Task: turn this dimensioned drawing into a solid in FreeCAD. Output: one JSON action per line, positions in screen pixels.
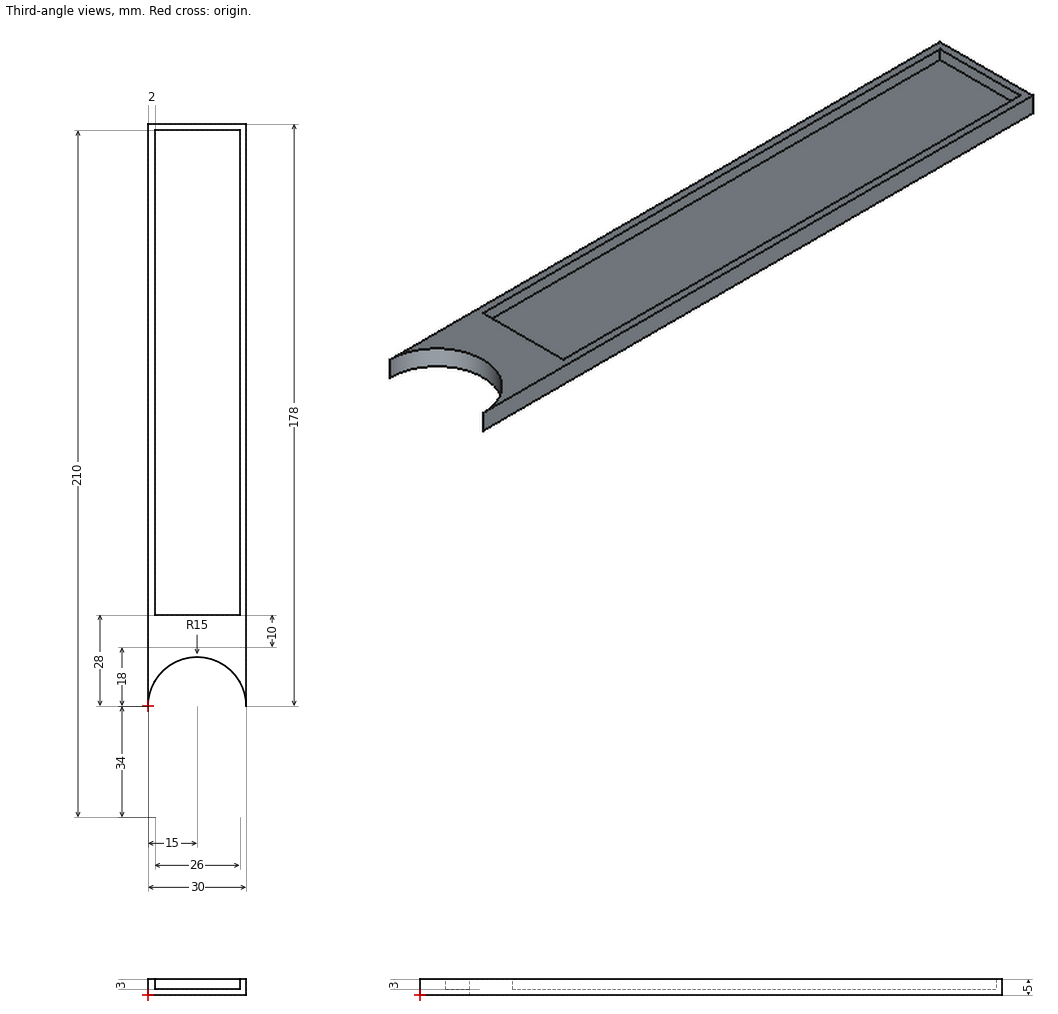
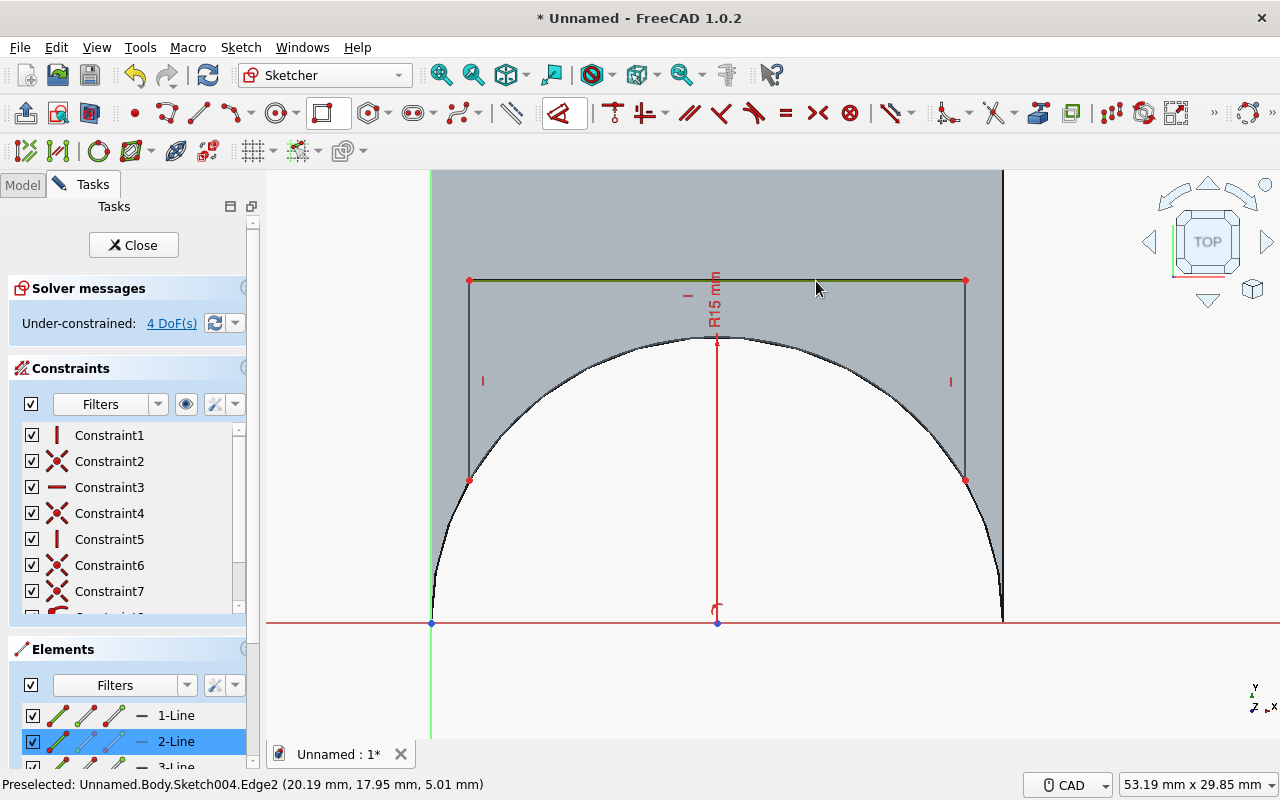
{"action": "key", "text": "l"}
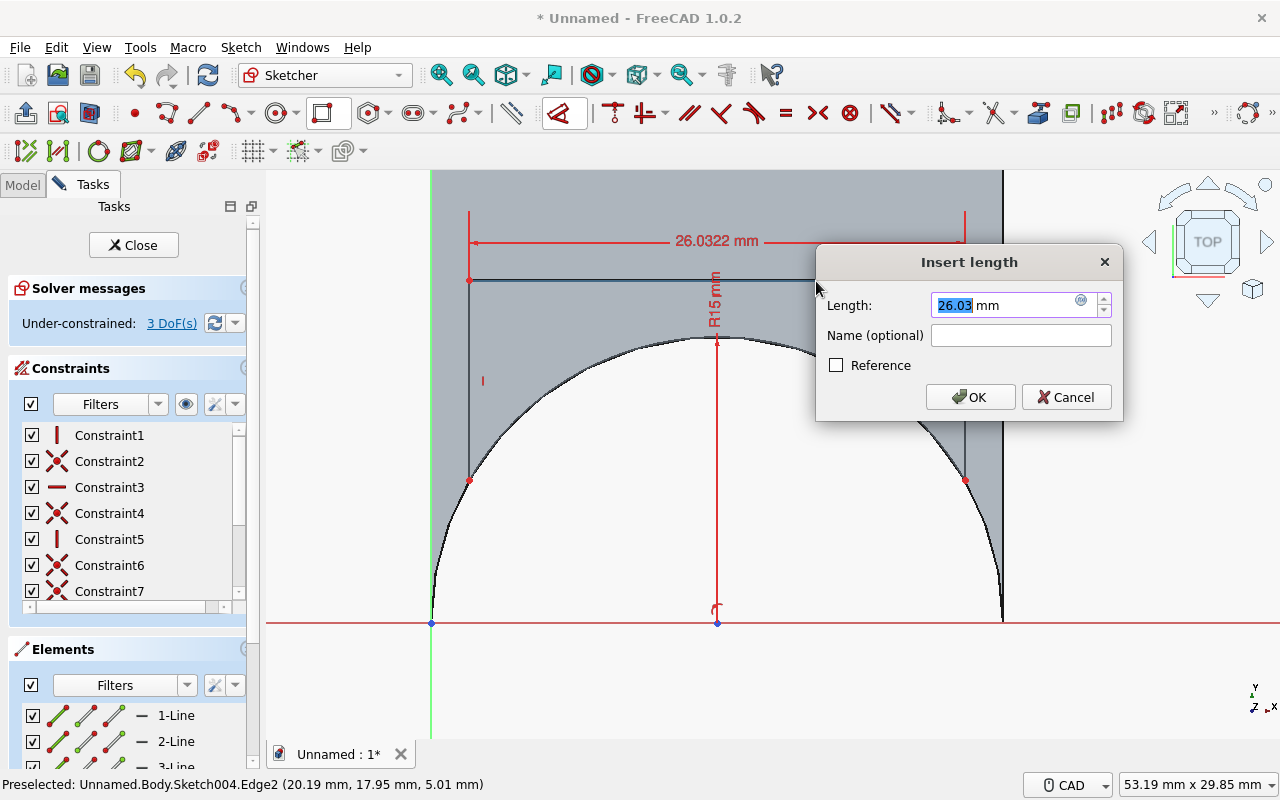
{"action": "type", "text": "26"}
{"action": "key", "text": "Return"}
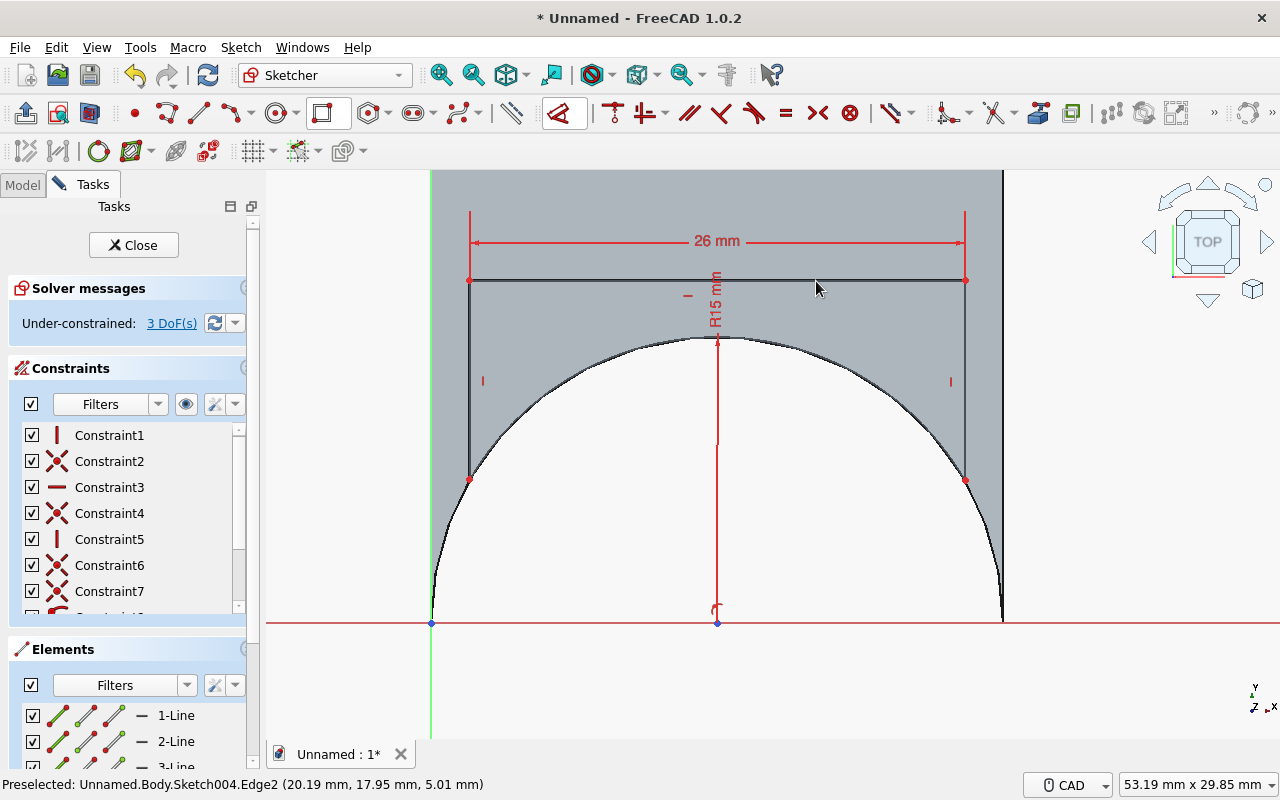
{"action": "left_click", "coordinate": [470, 281]}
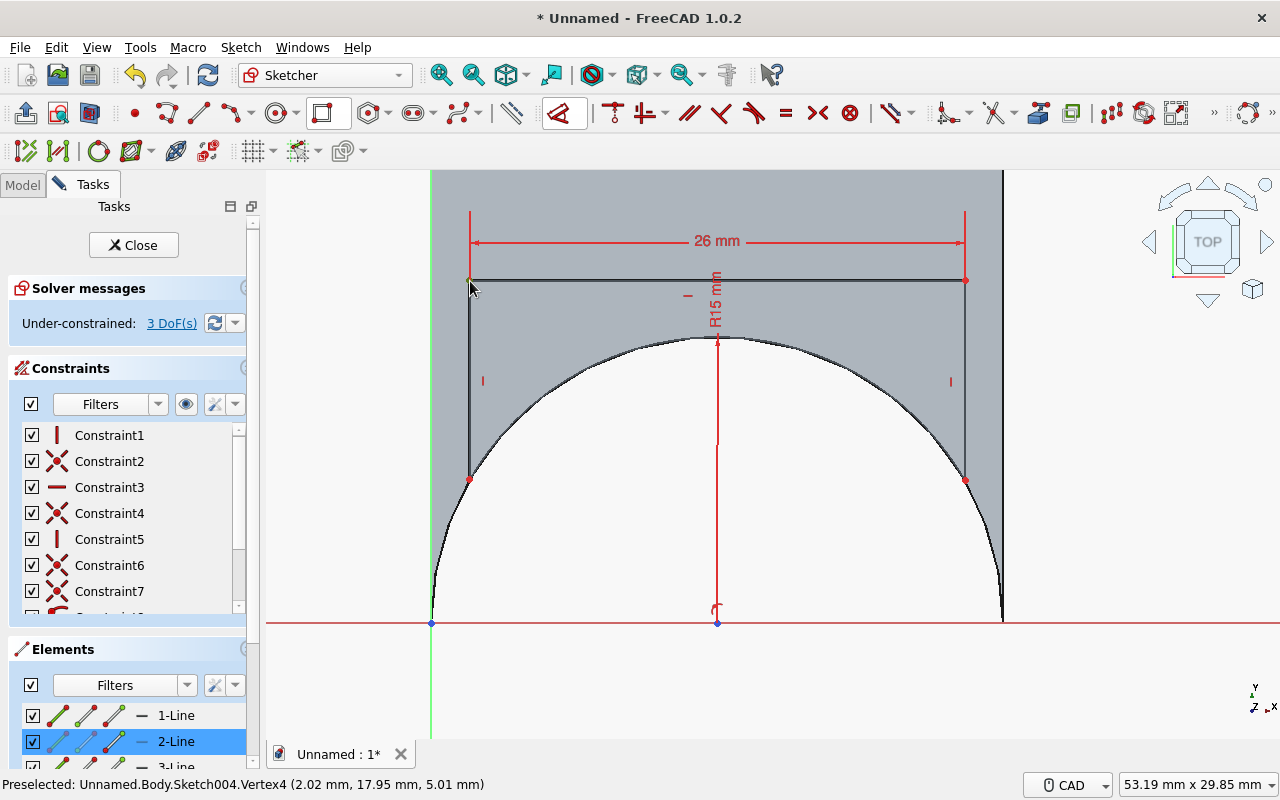
{"action": "key", "text": "l"}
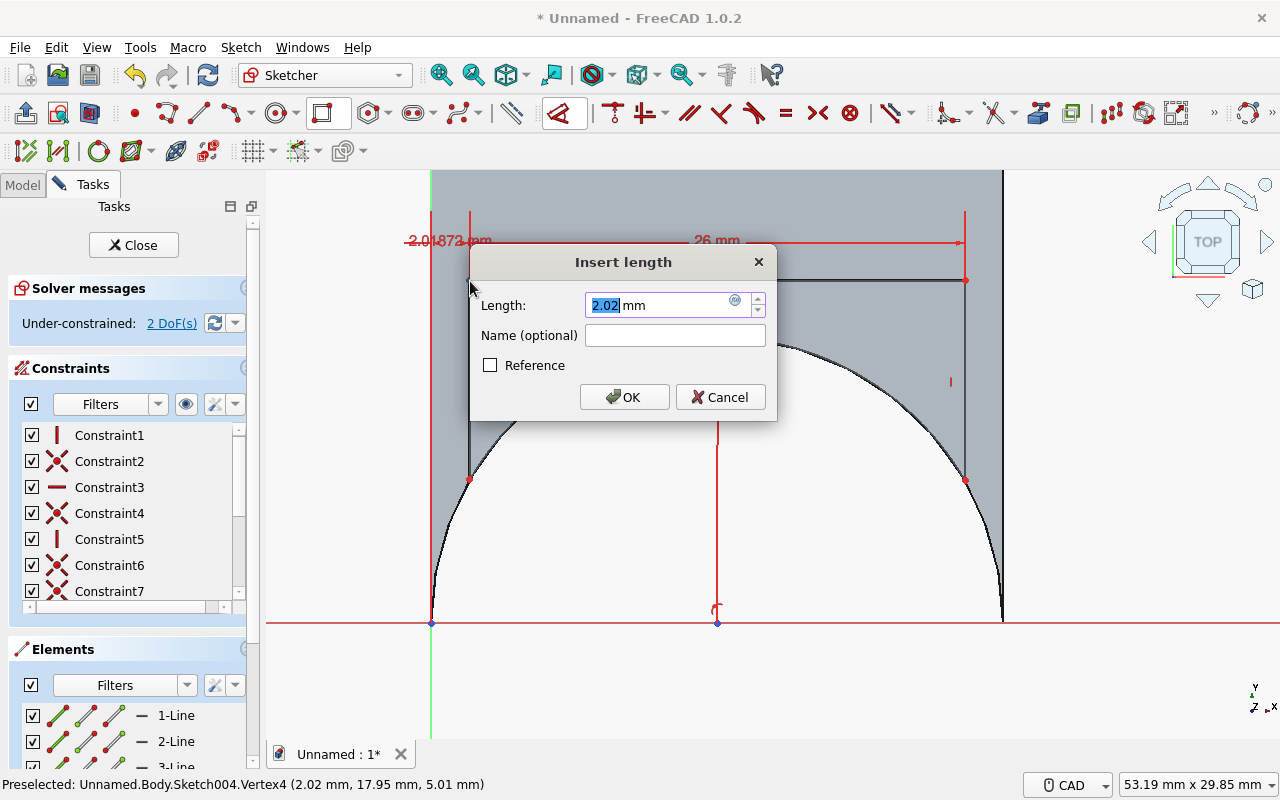
{"action": "type", "text": "2"}
{"action": "key", "text": "Return"}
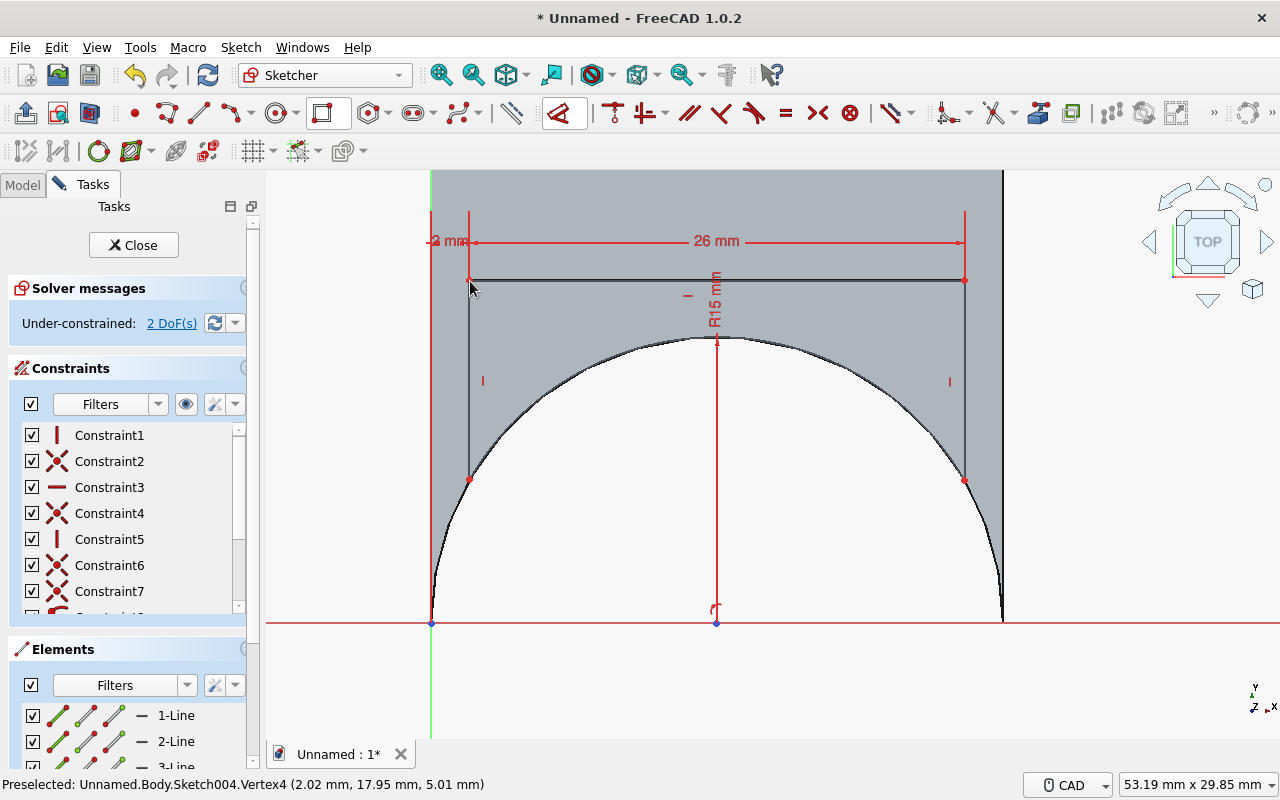
{"action": "left_click", "coordinate": [965, 281]}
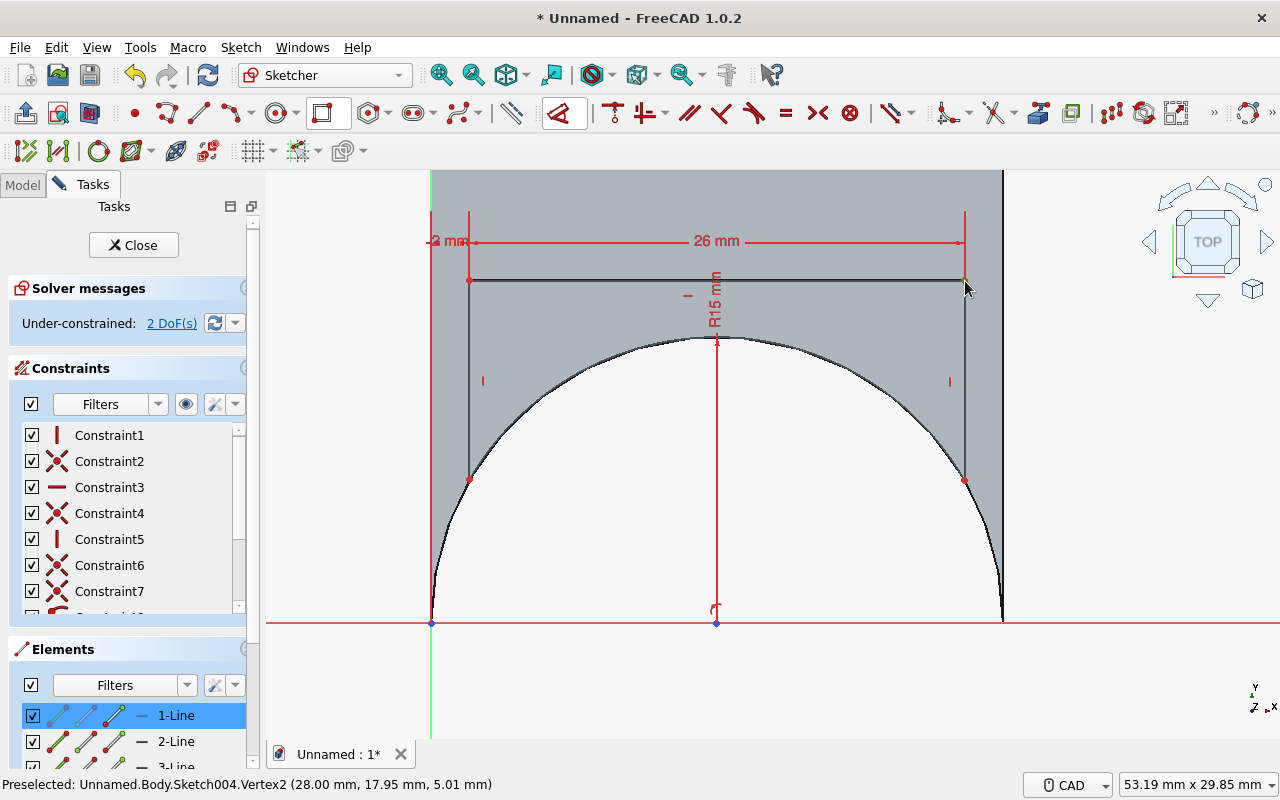
{"action": "key", "text": "i"}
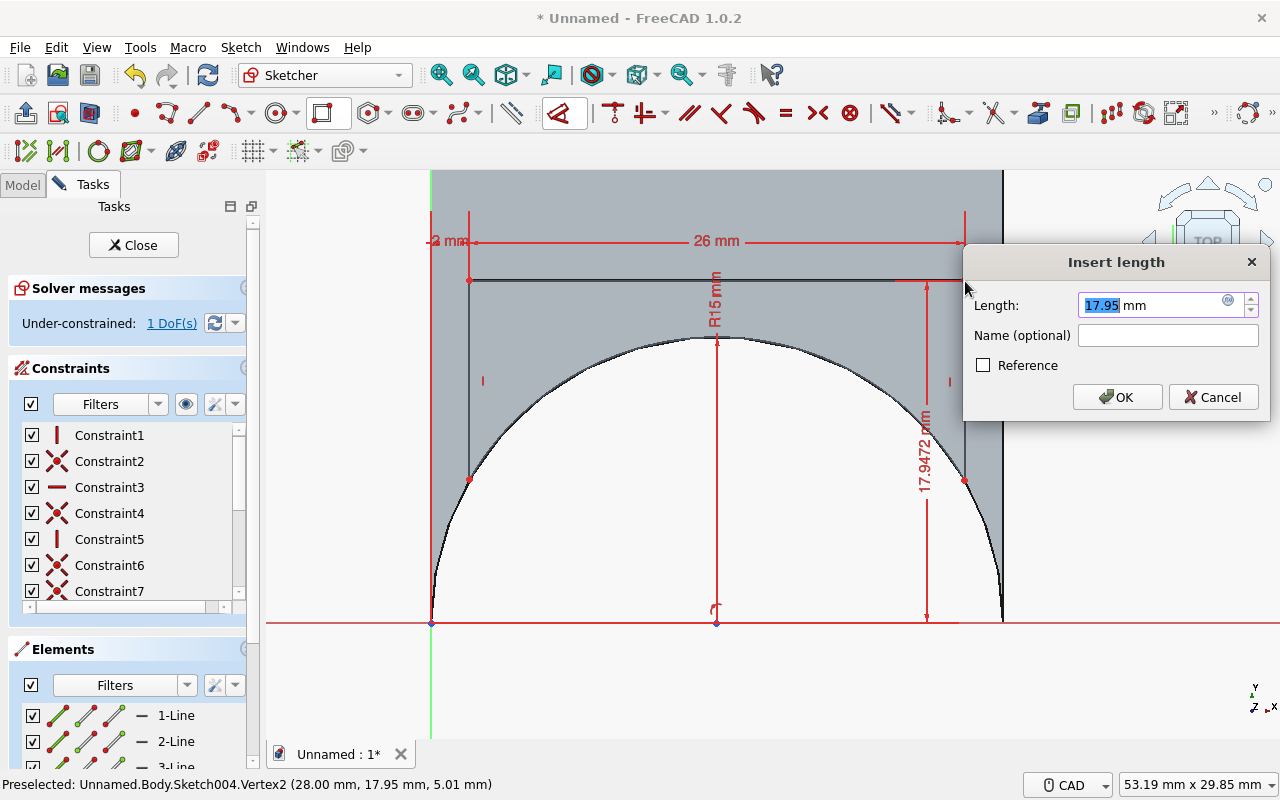
{"action": "type", "text": "18"}
{"action": "key", "text": "Return"}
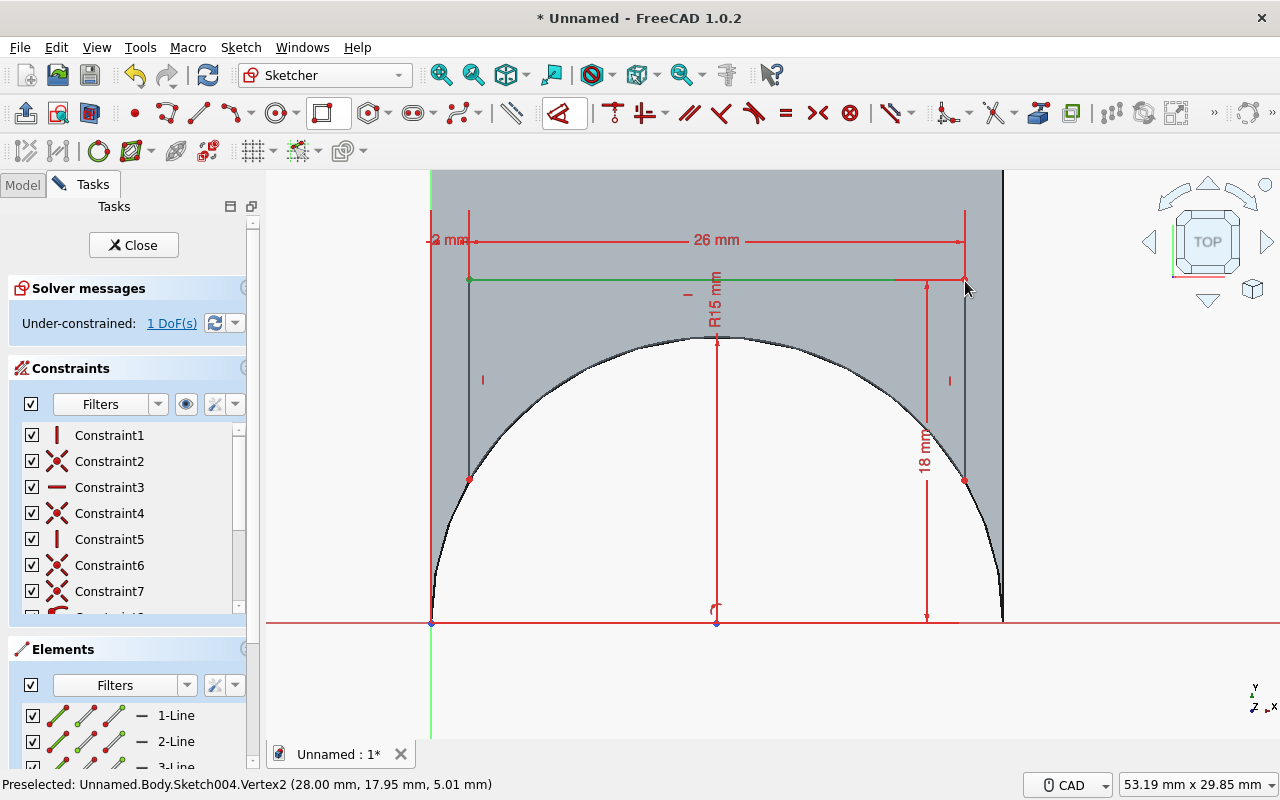
{"action": "left_click", "coordinate": [717, 623]}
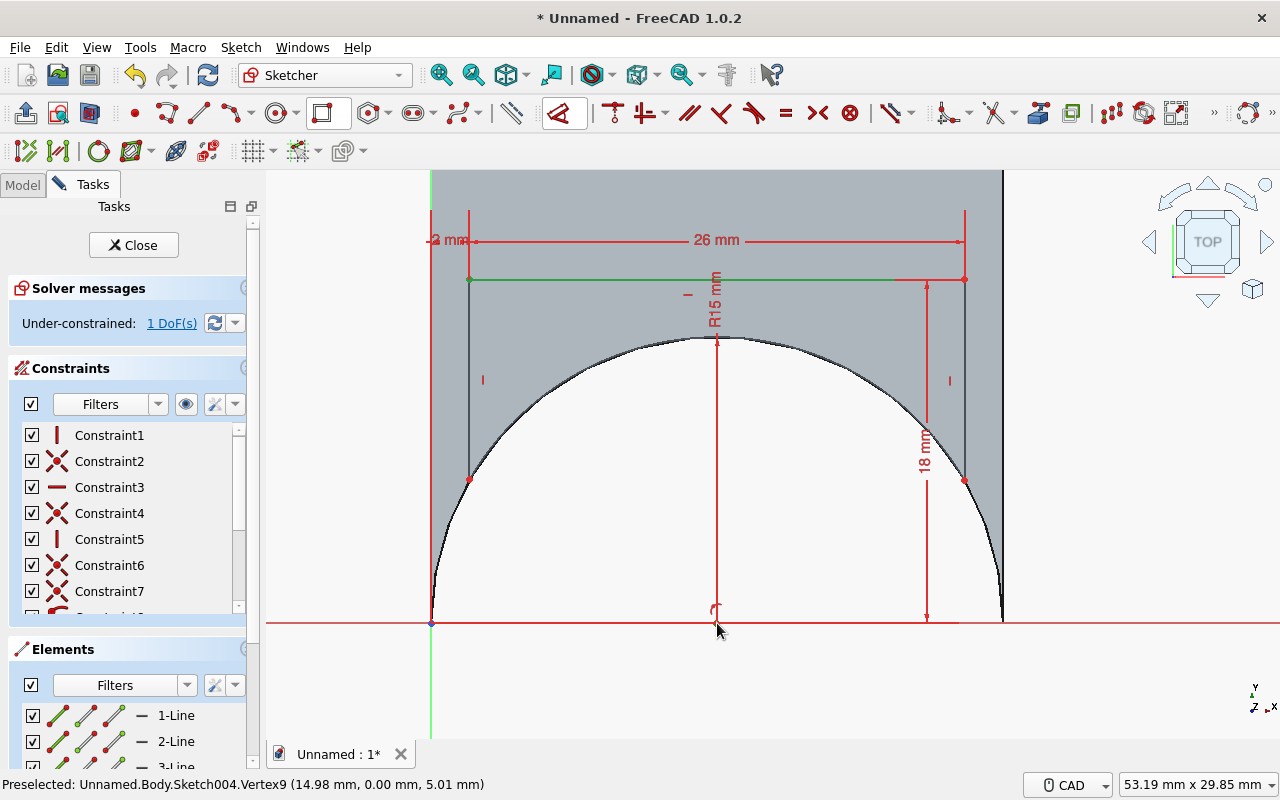
{"action": "key", "text": "l"}